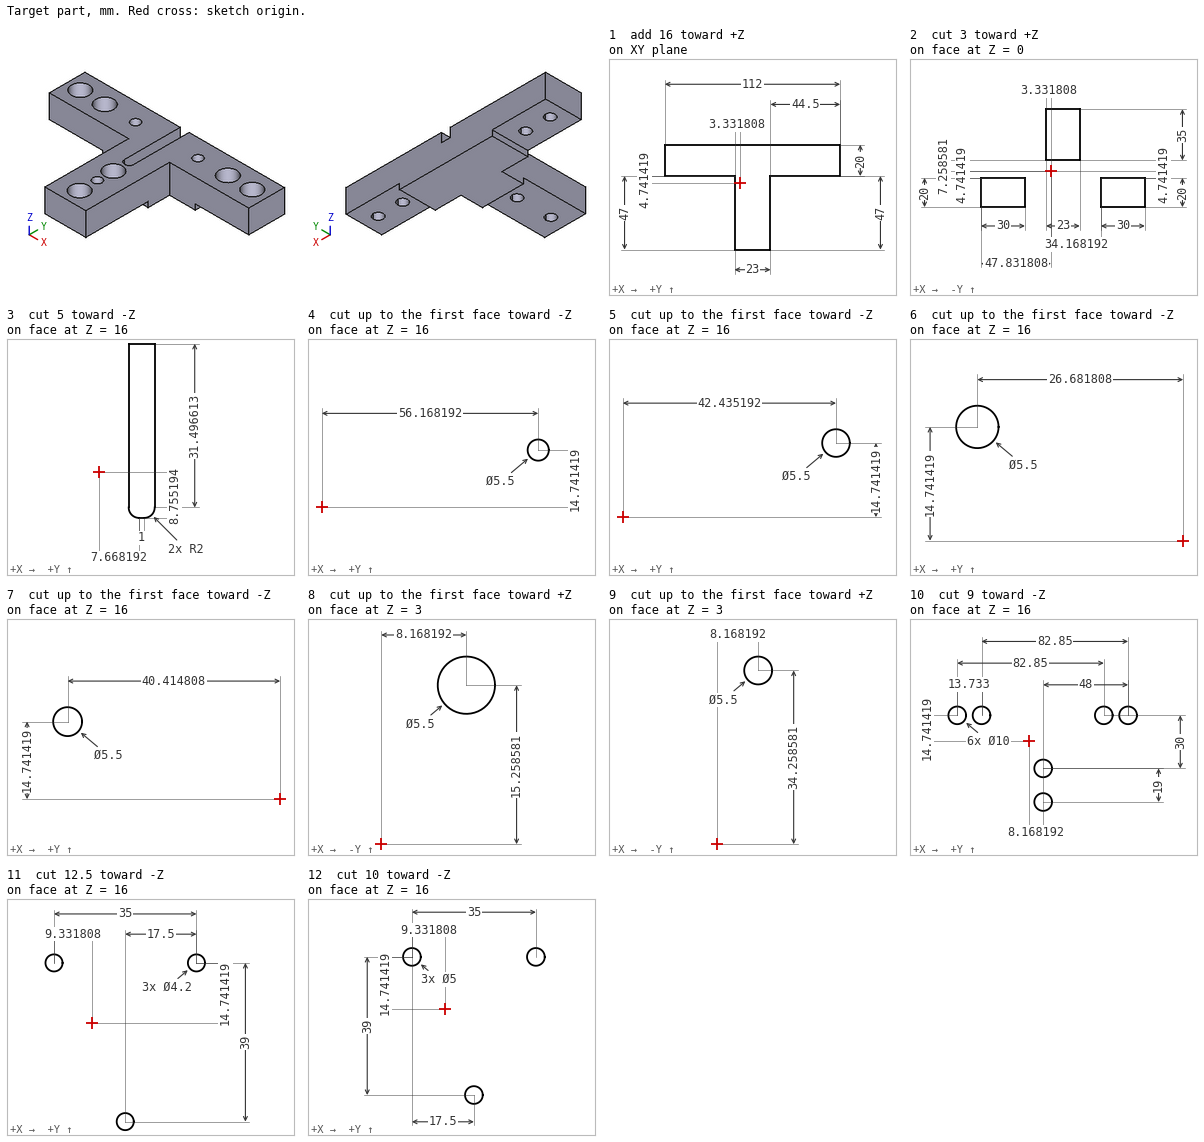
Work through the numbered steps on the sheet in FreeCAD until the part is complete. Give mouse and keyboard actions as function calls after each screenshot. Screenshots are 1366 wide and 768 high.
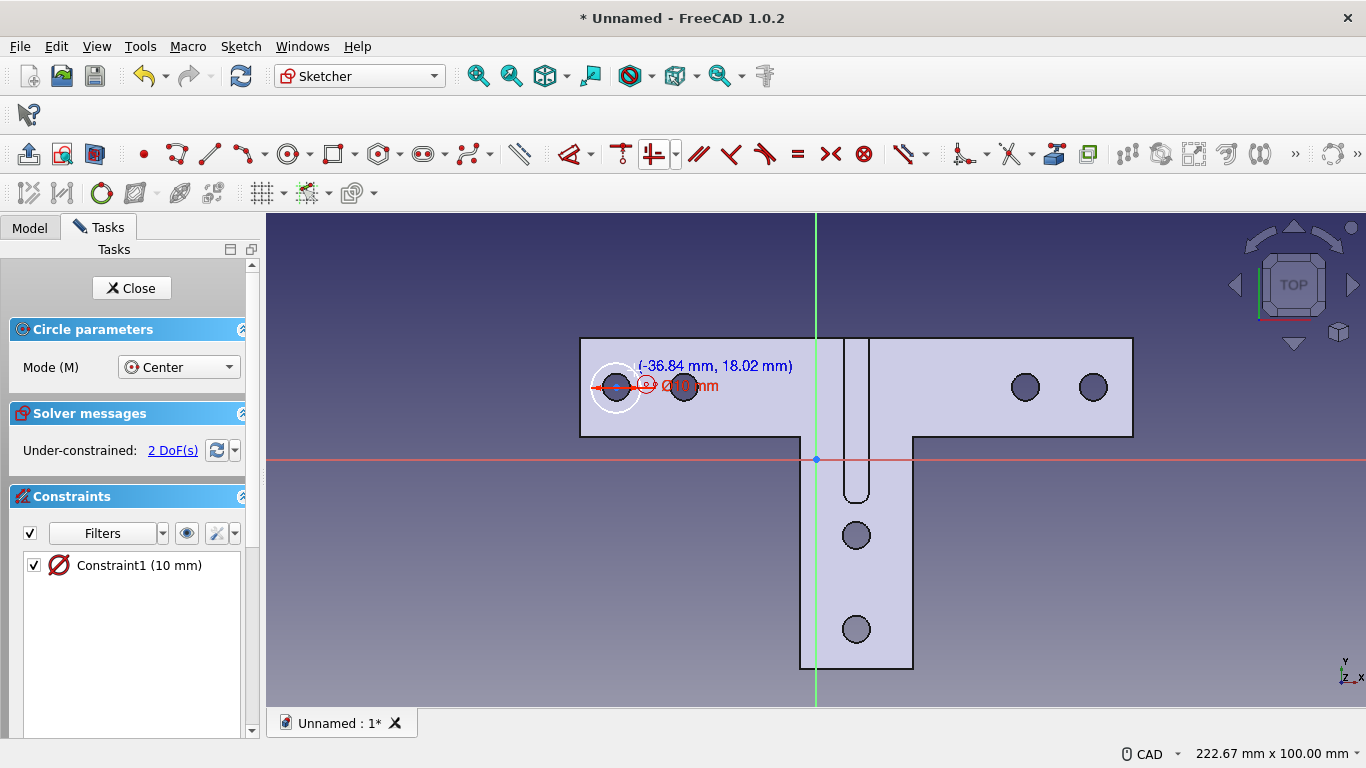
click(684, 387)
move(702, 370)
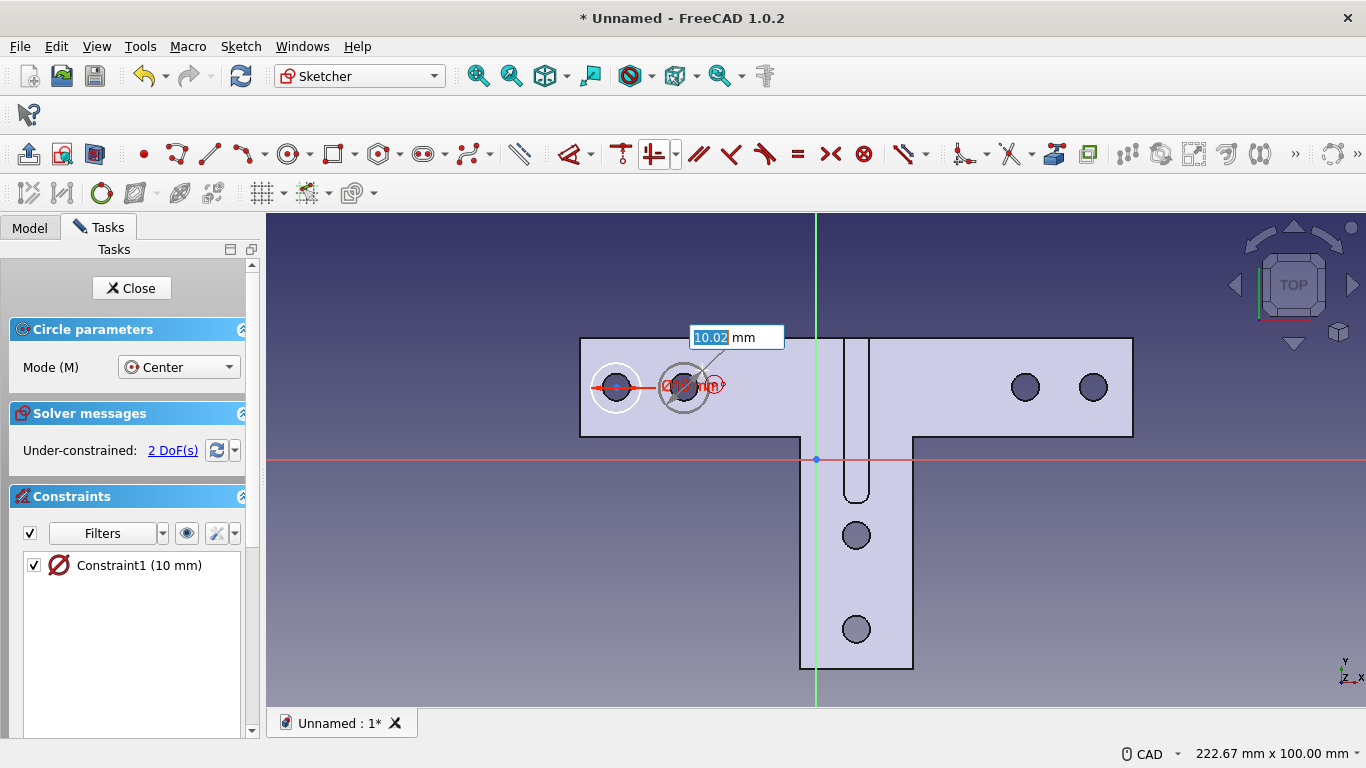
text(10)
key(Return)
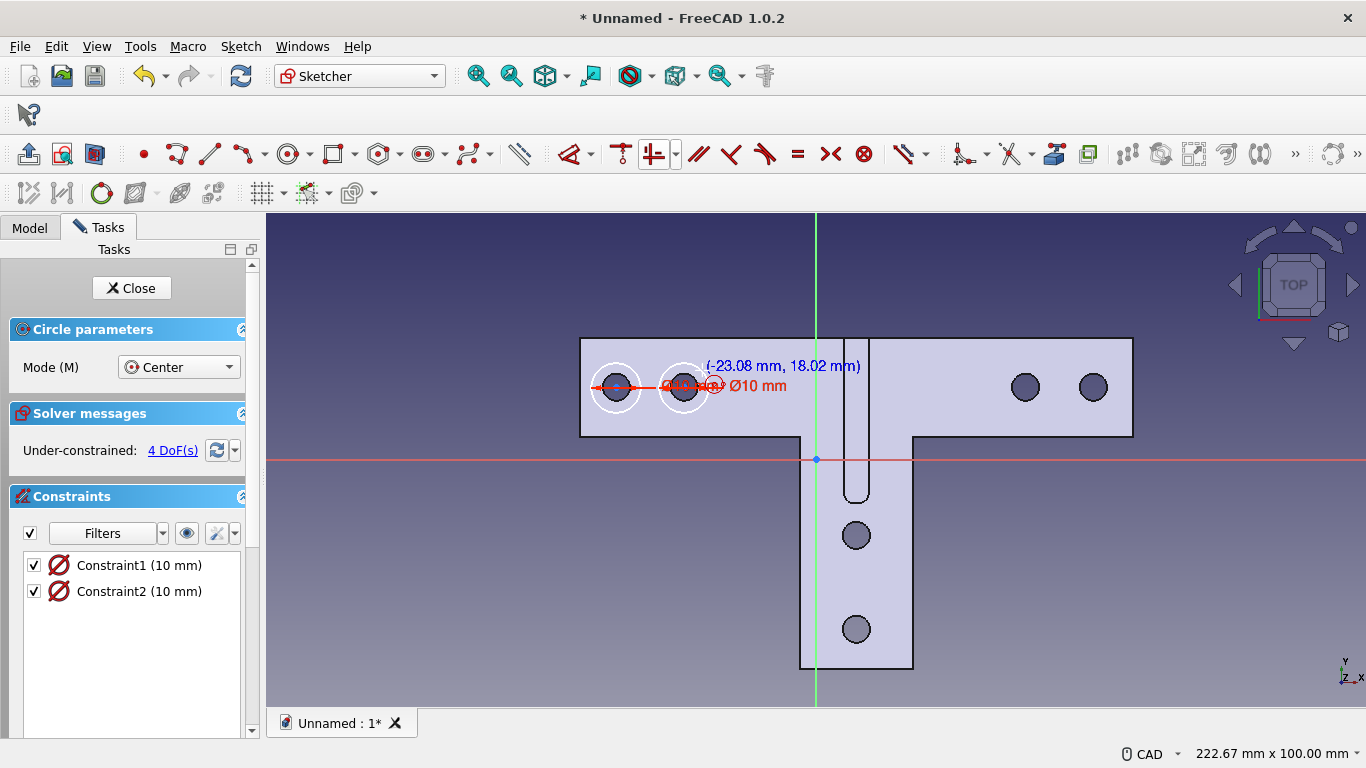
click(1026, 387)
move(1043, 370)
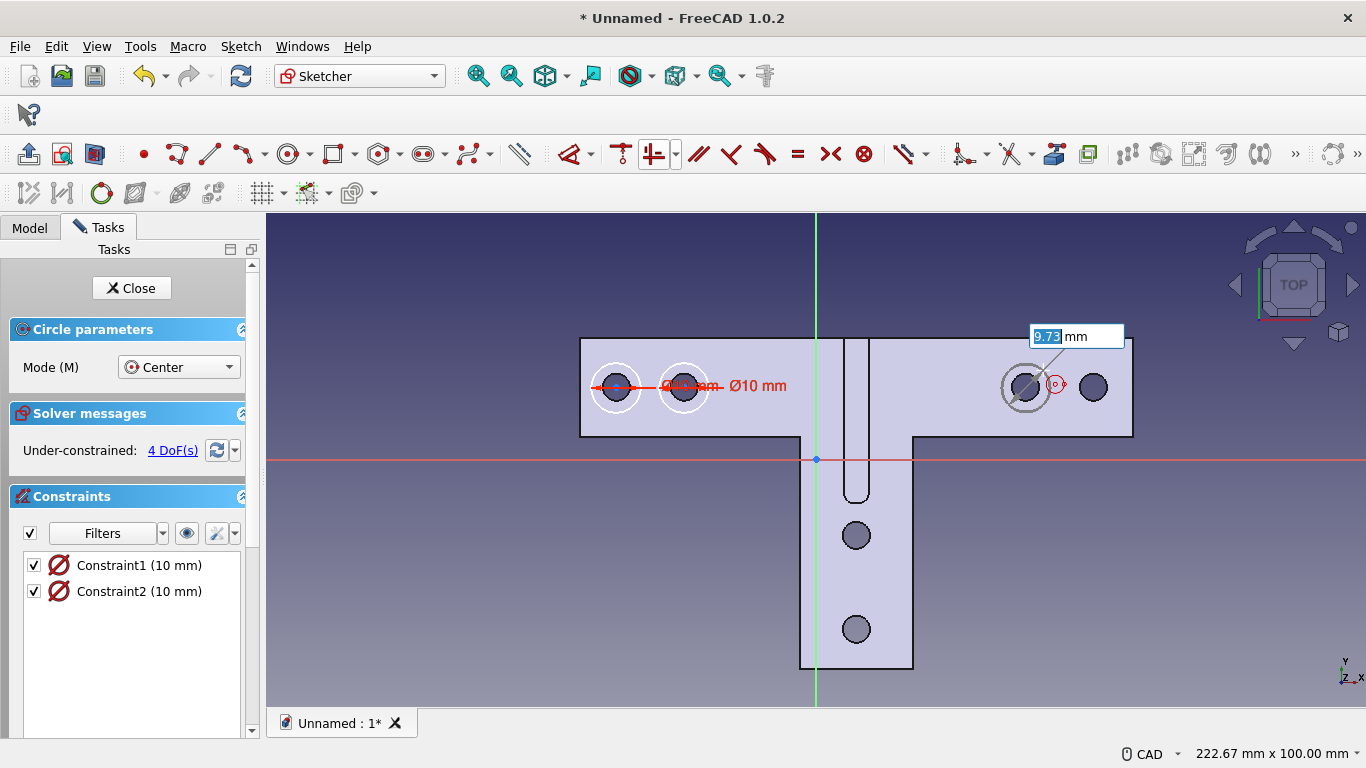
text(10)
key(Return)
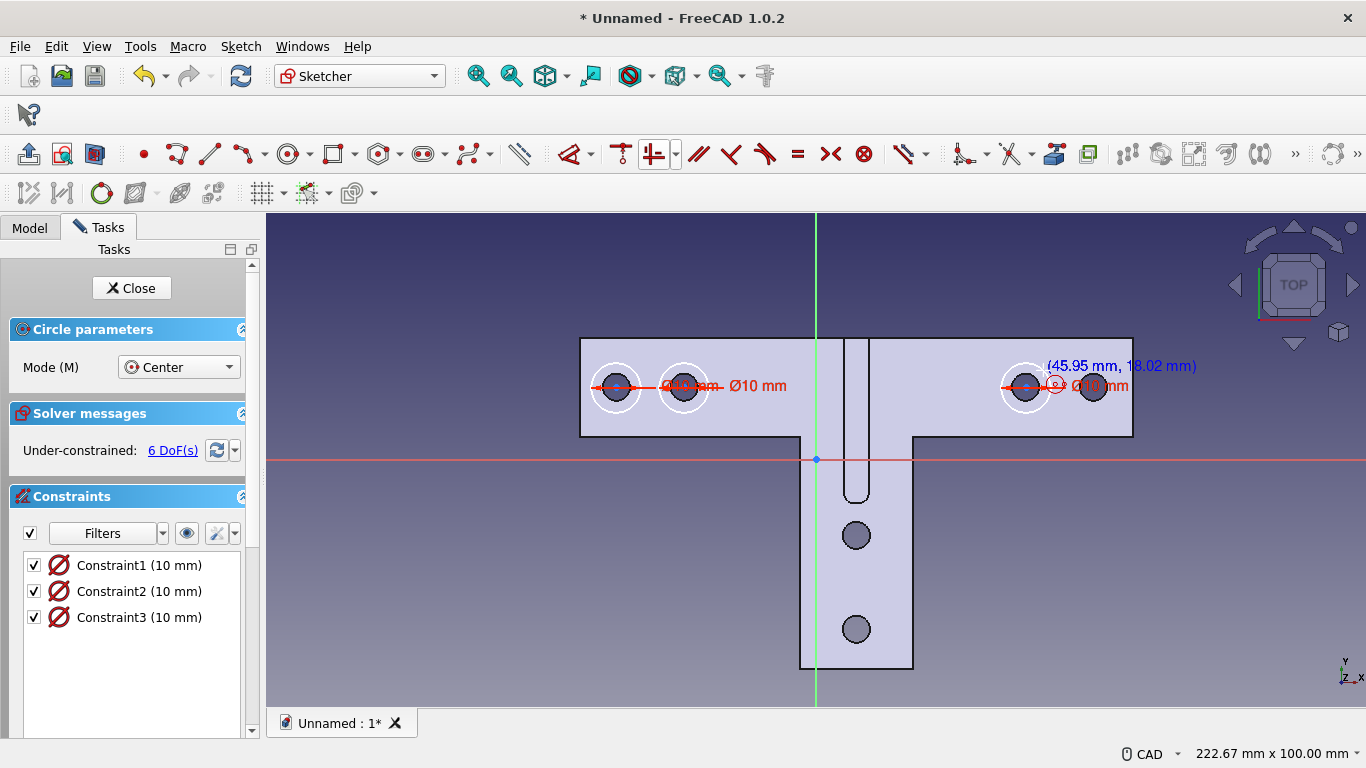
click(1093, 387)
move(1111, 370)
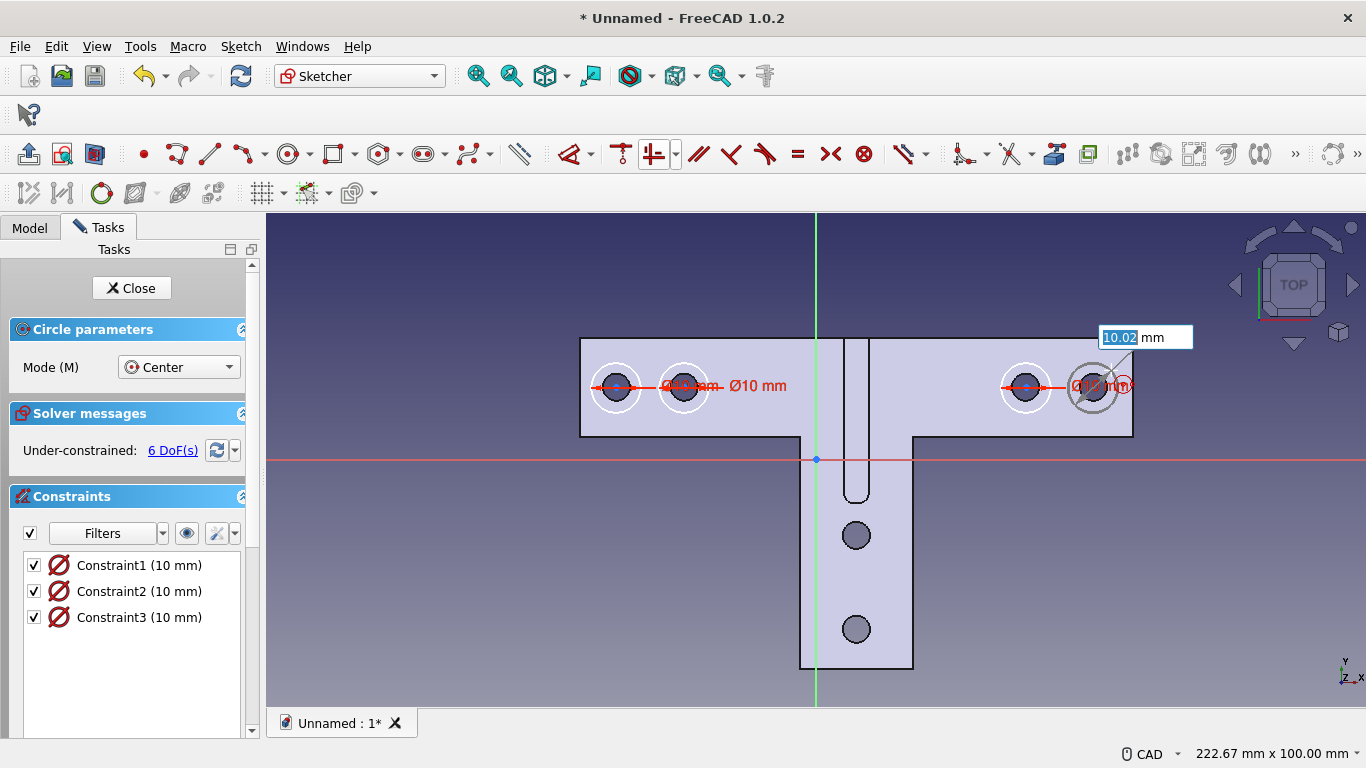
text(10)
key(Return)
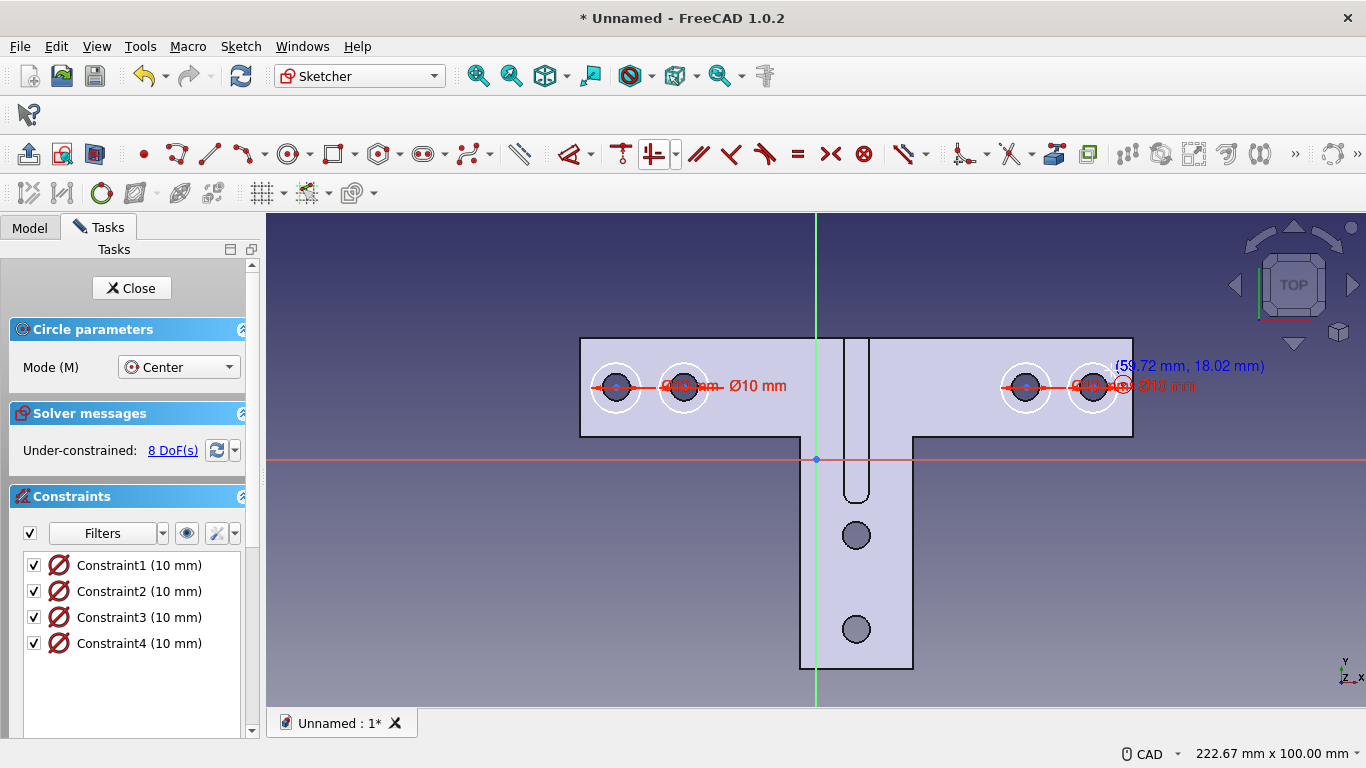
click(856, 535)
move(874, 518)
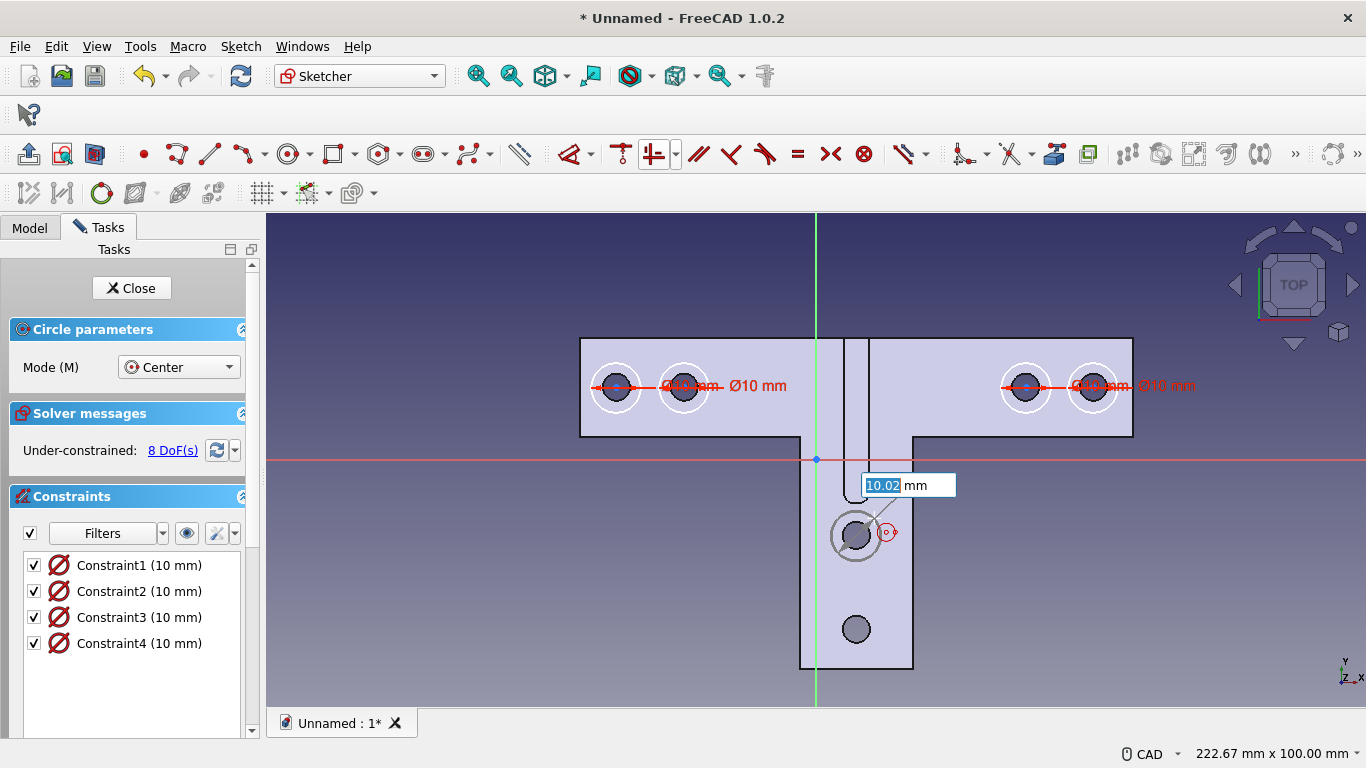
text(10)
key(Return)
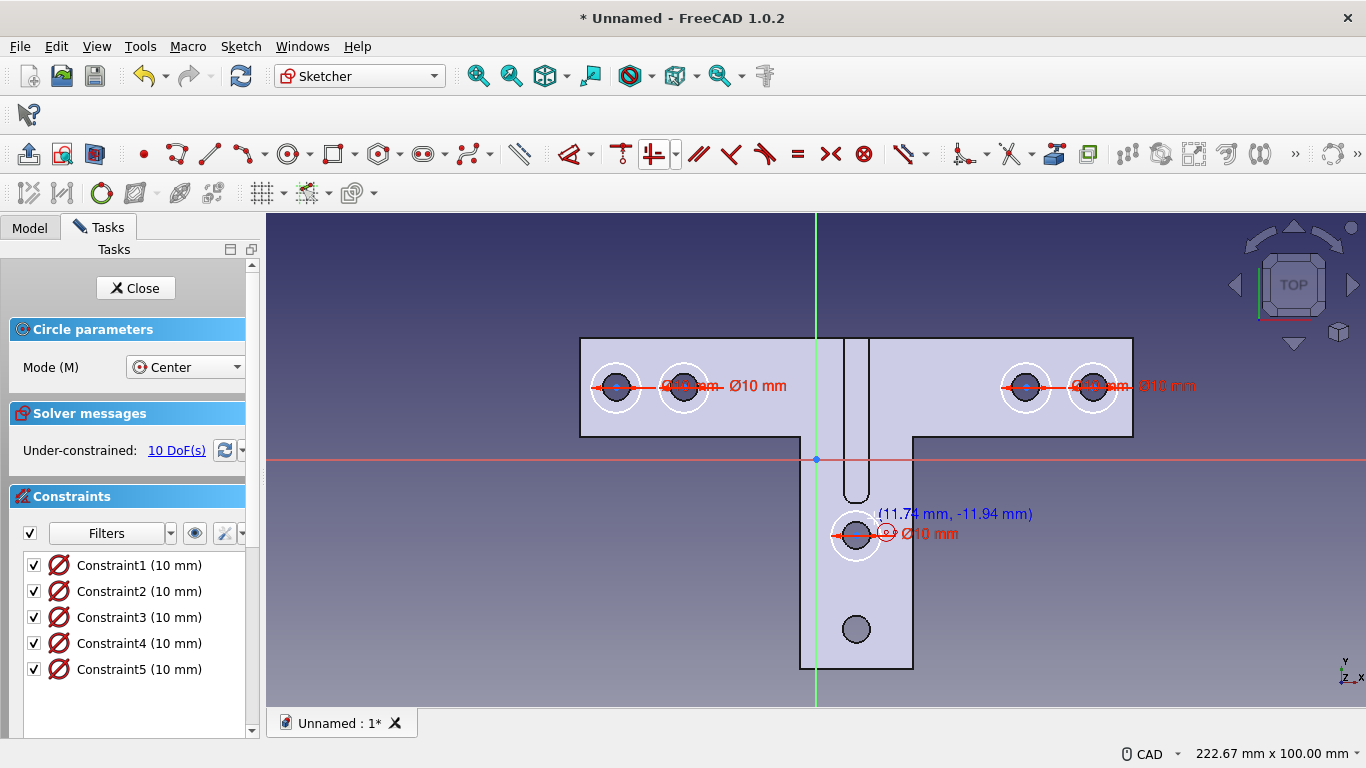
click(856, 629)
move(874, 612)